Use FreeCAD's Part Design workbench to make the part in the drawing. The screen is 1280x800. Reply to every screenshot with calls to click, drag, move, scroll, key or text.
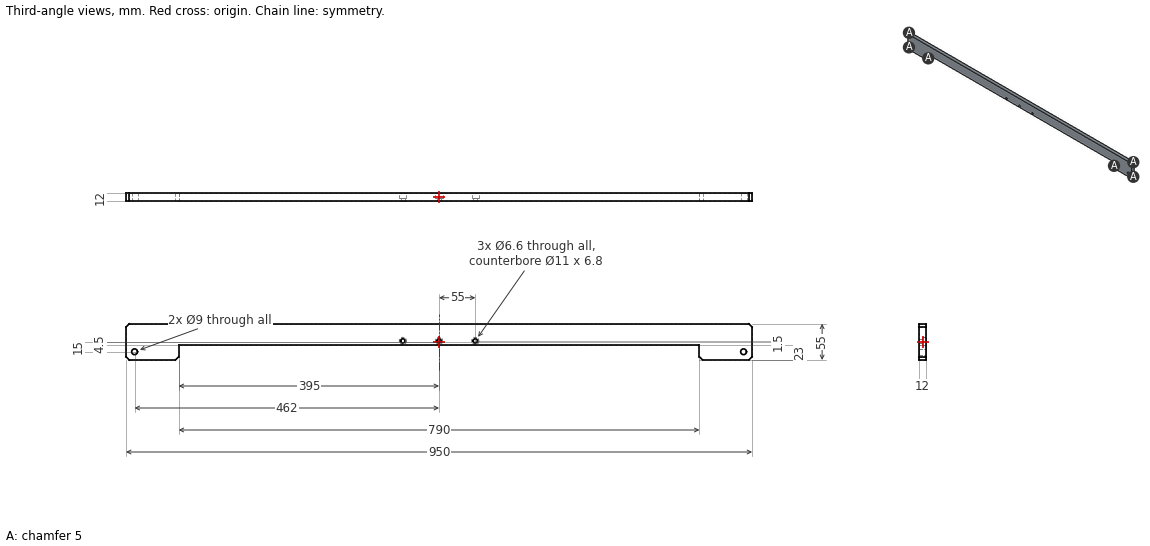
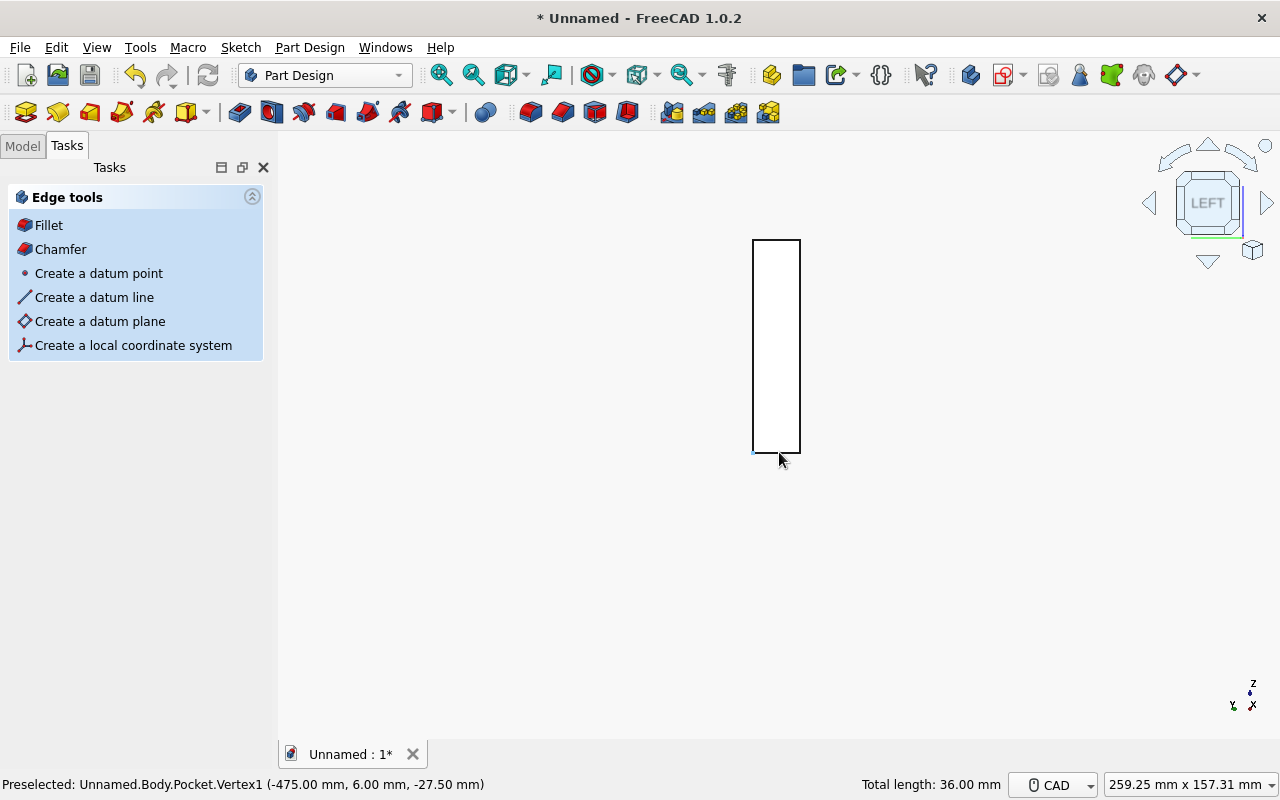
click(776, 239, ctrl)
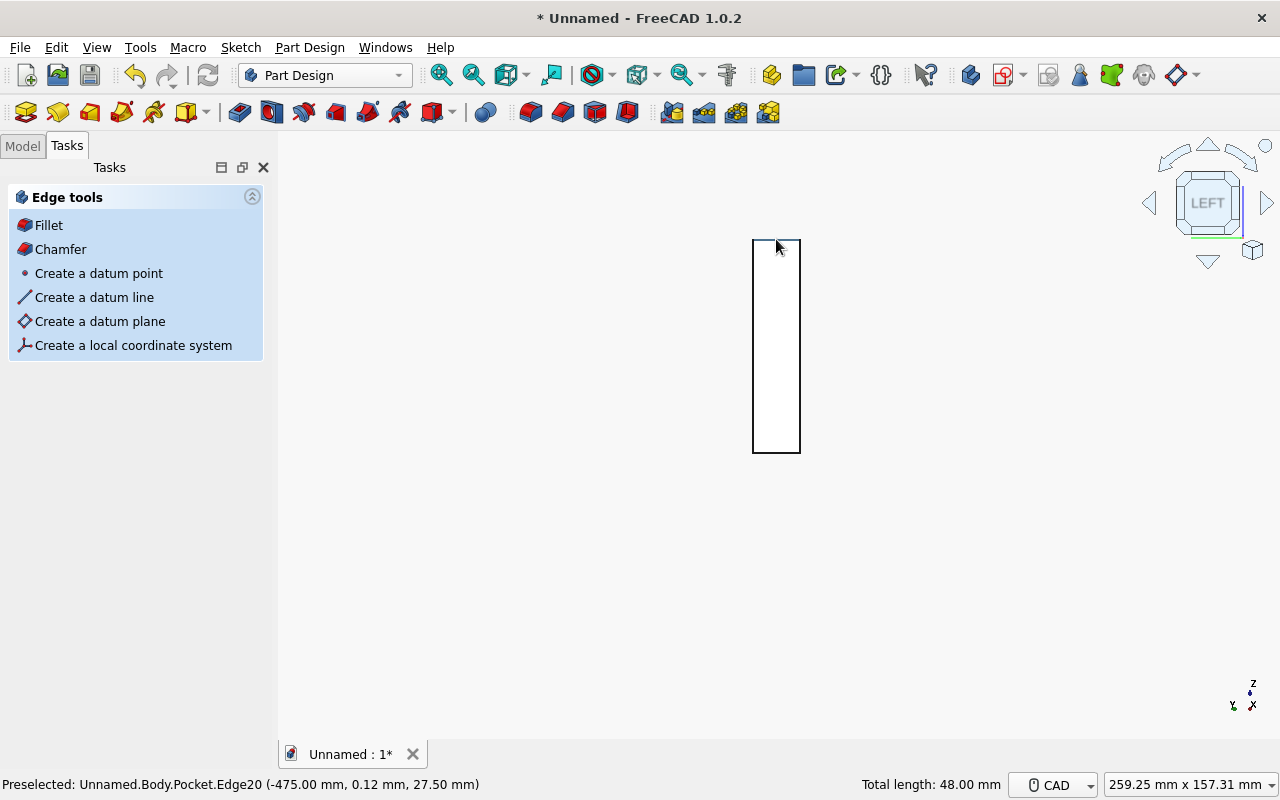
click(776, 452, ctrl)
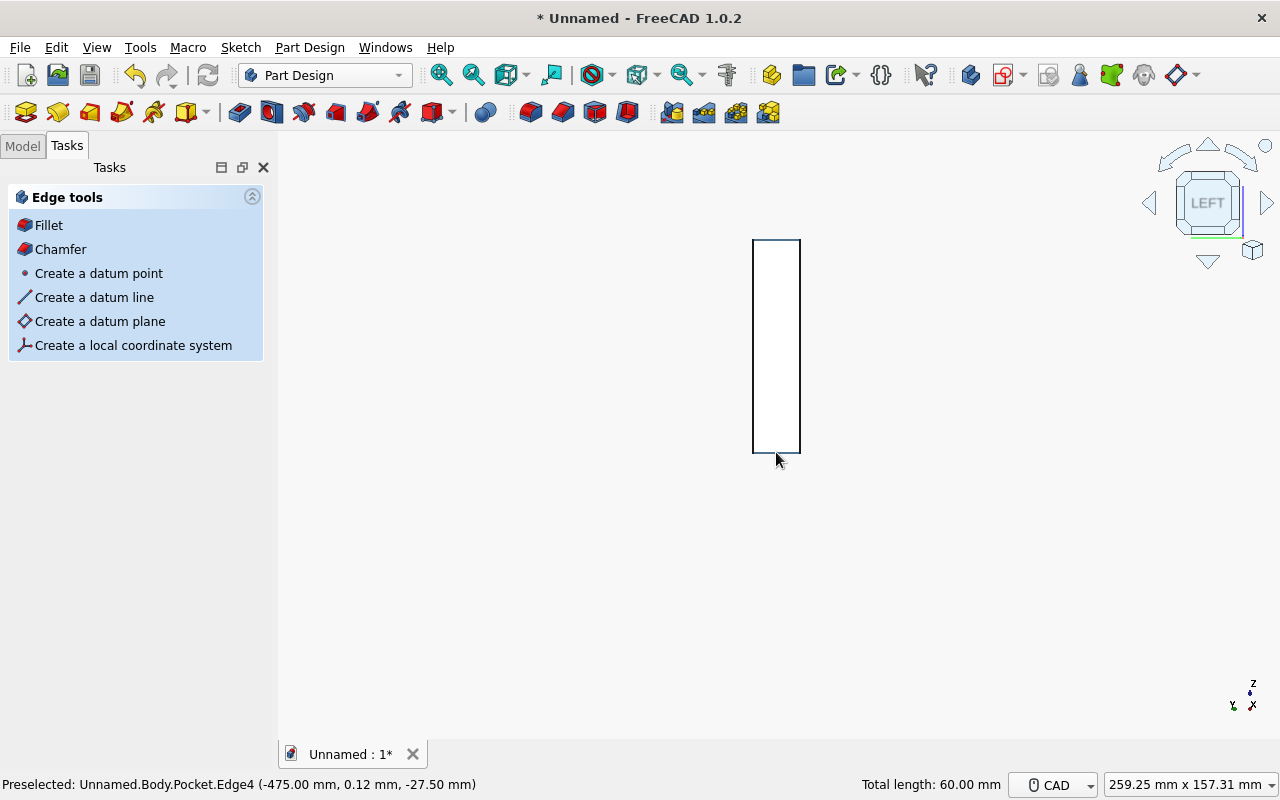
key(v)
key(f)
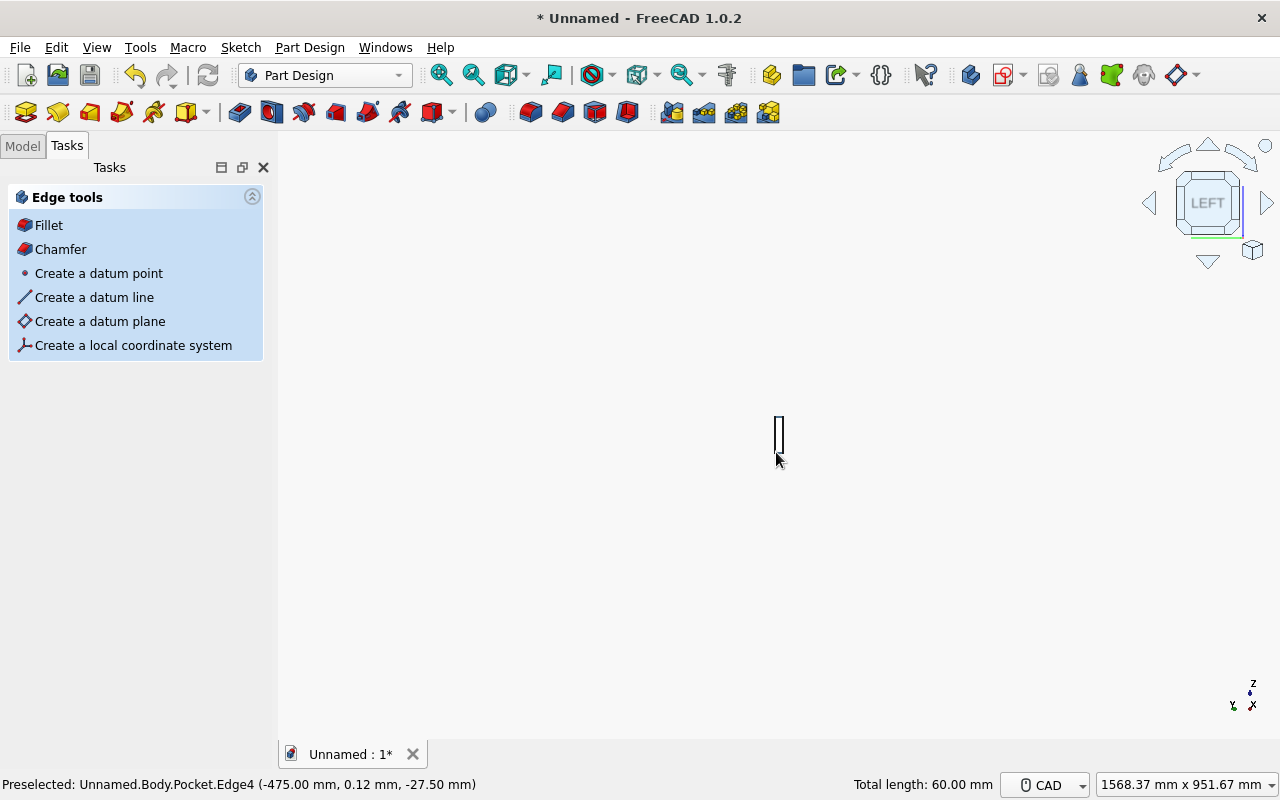
key(v)
key(3)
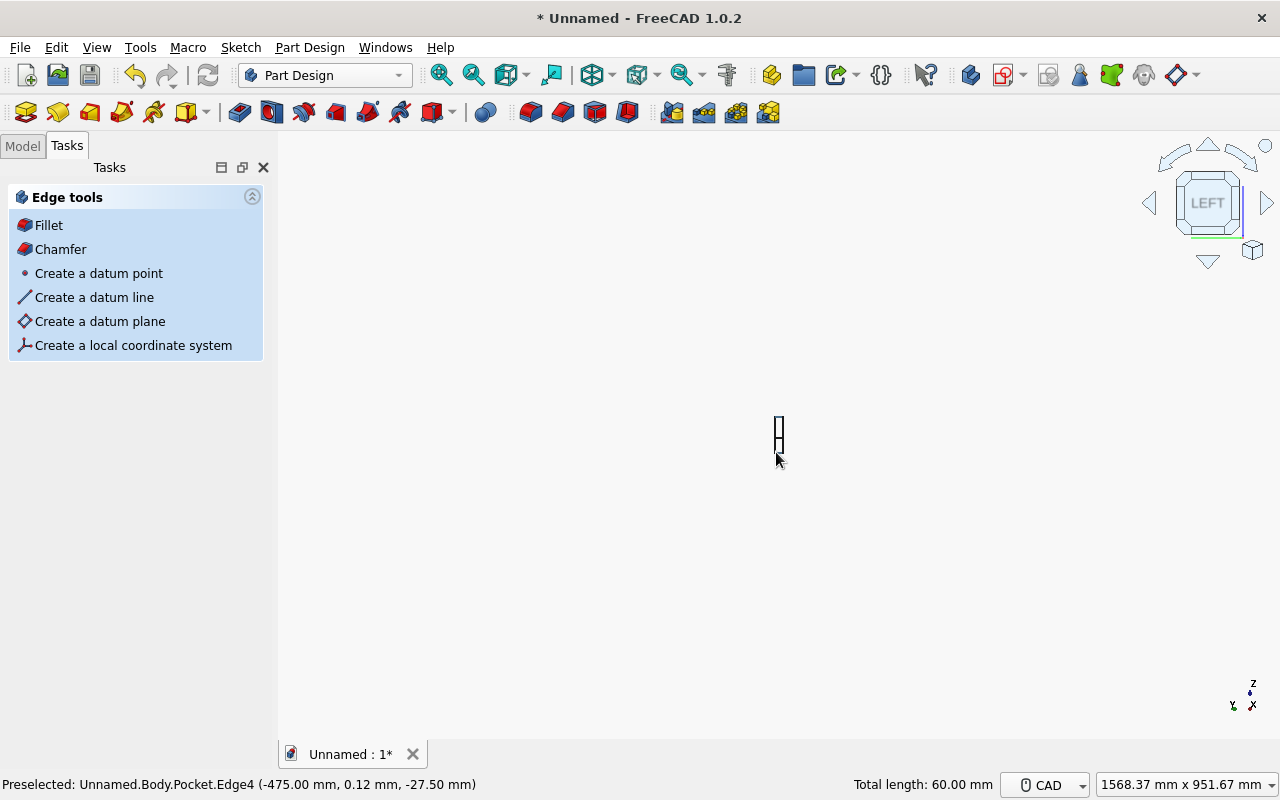
key(0)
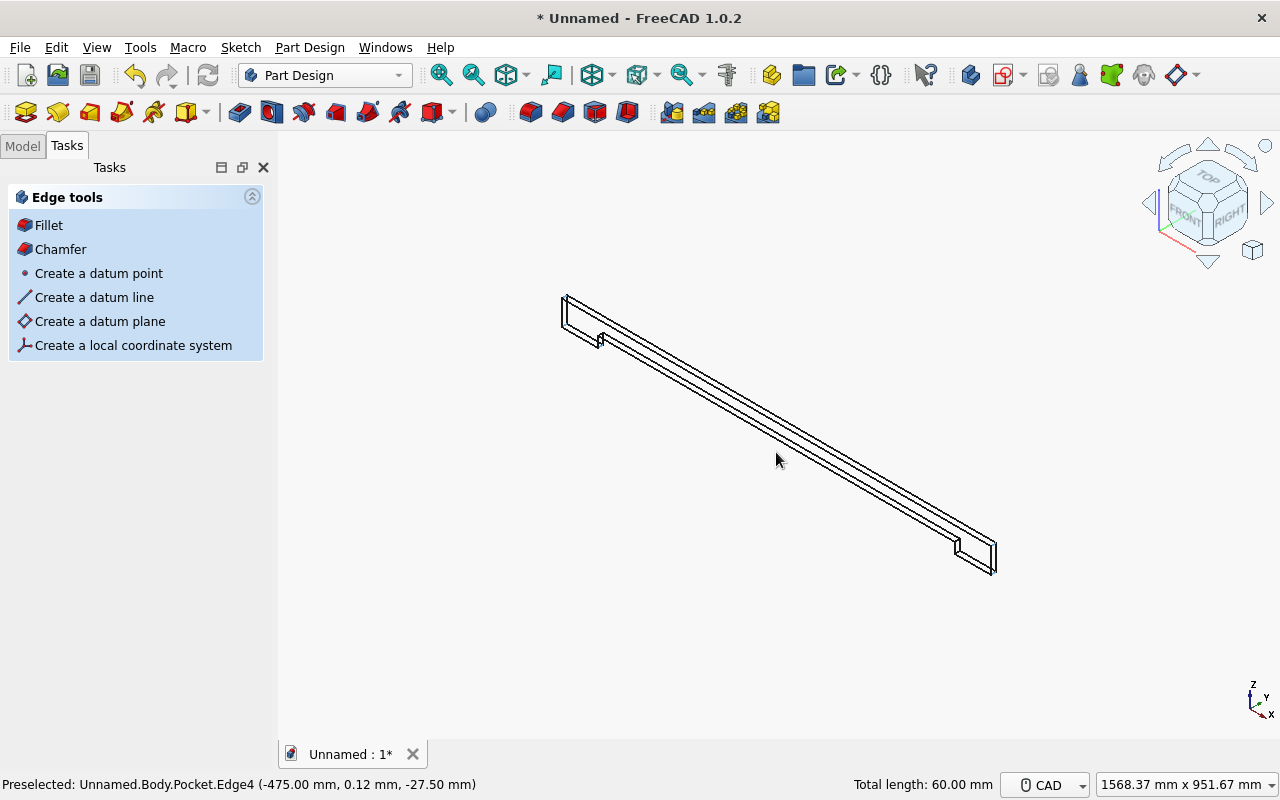
scroll(957, 551, up, 9)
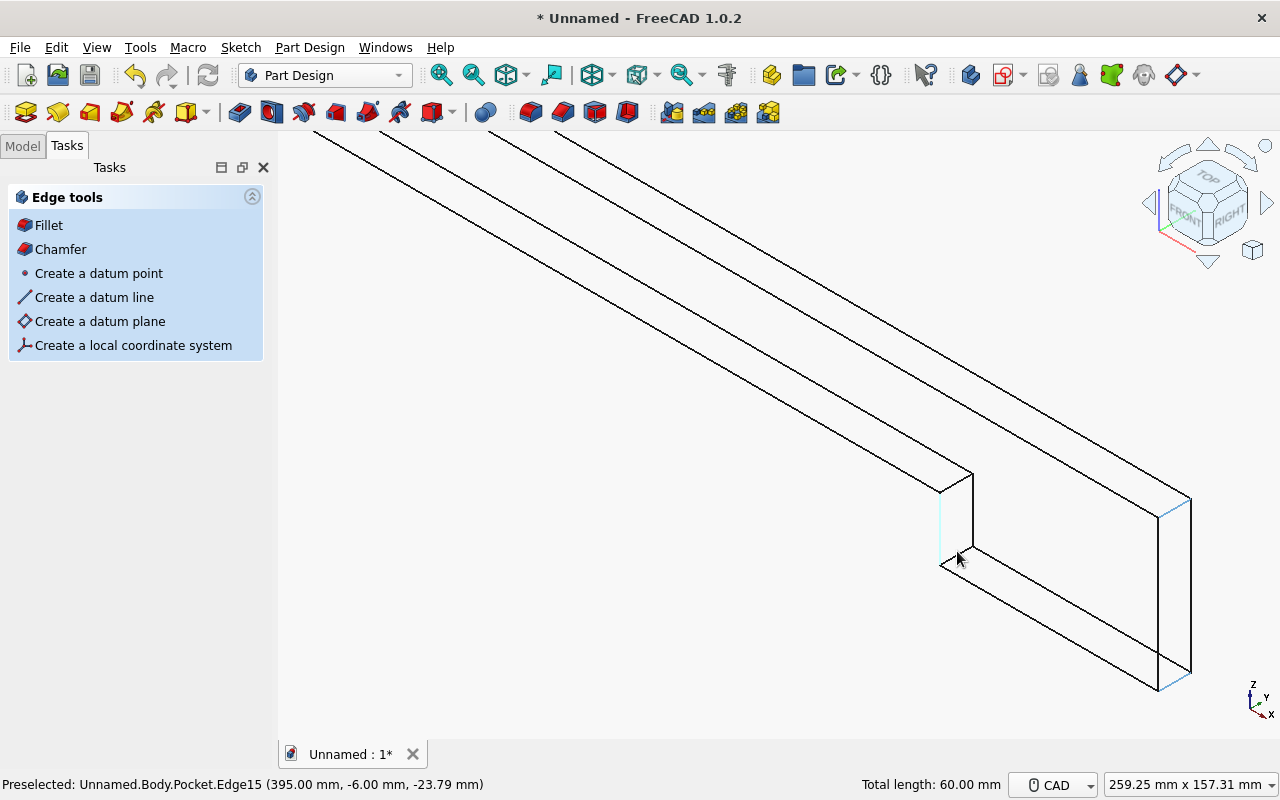
click(956, 555, ctrl)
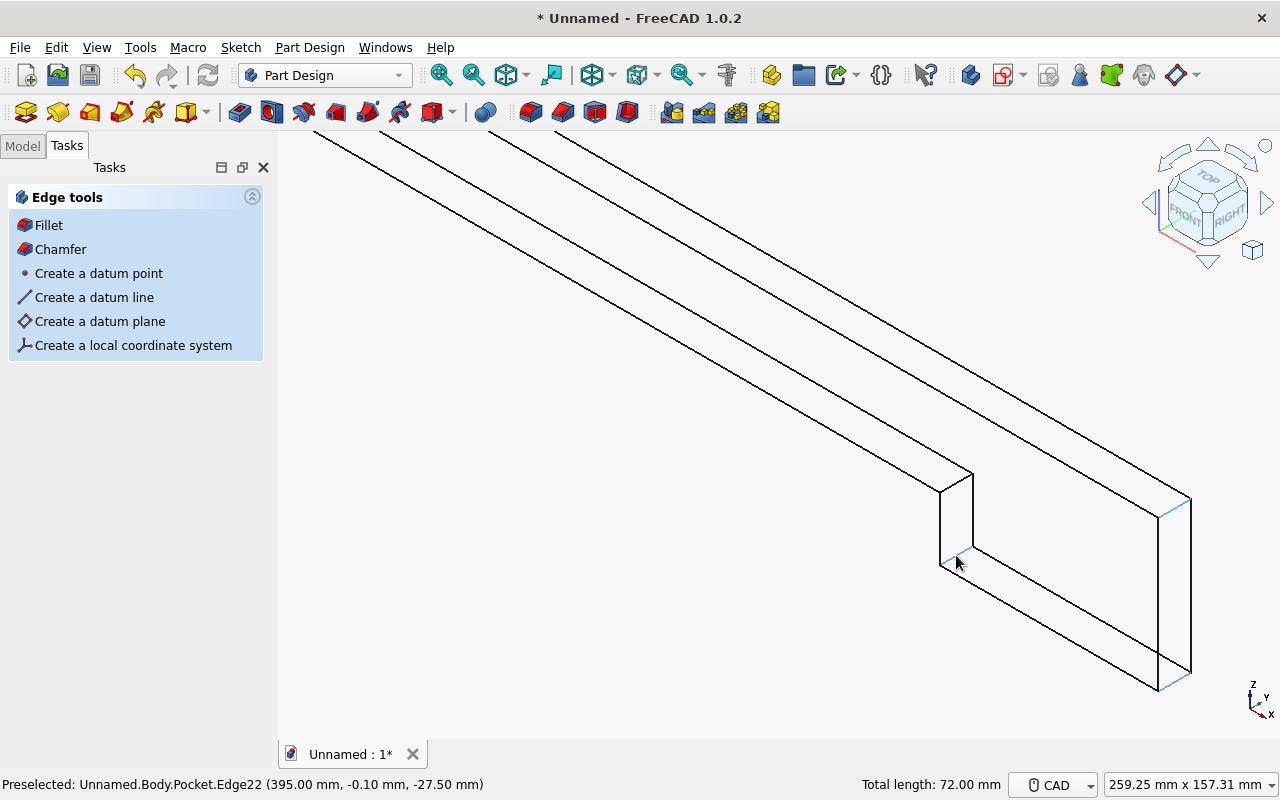
key(v)
key(1)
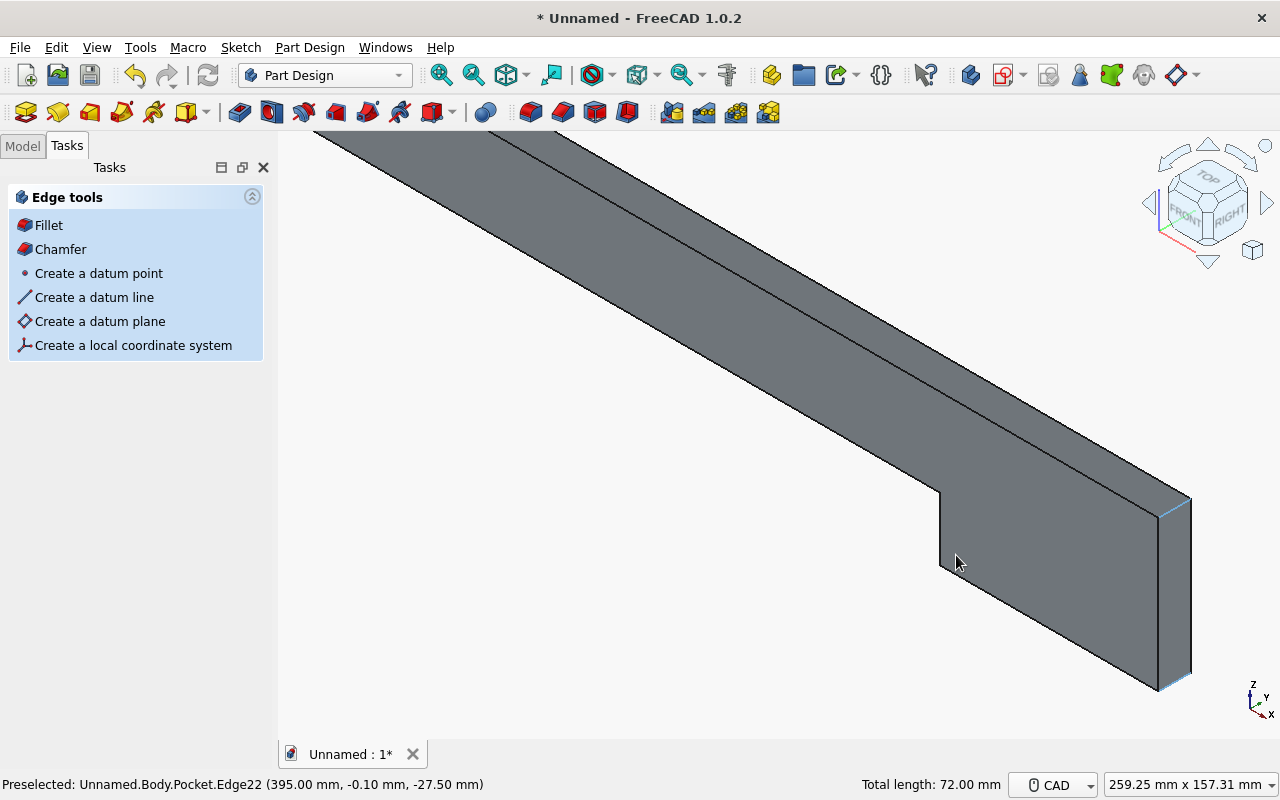
click(564, 112)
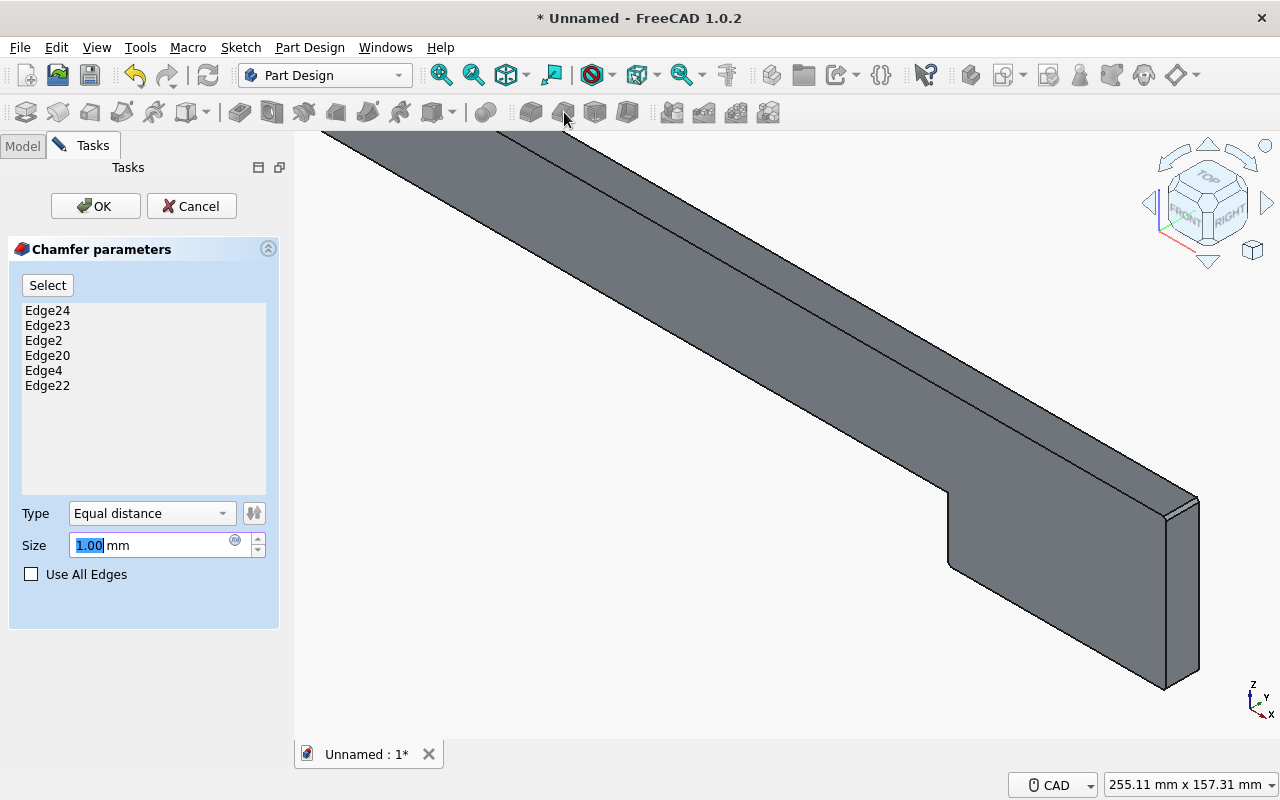
text(5)
key(Tab)